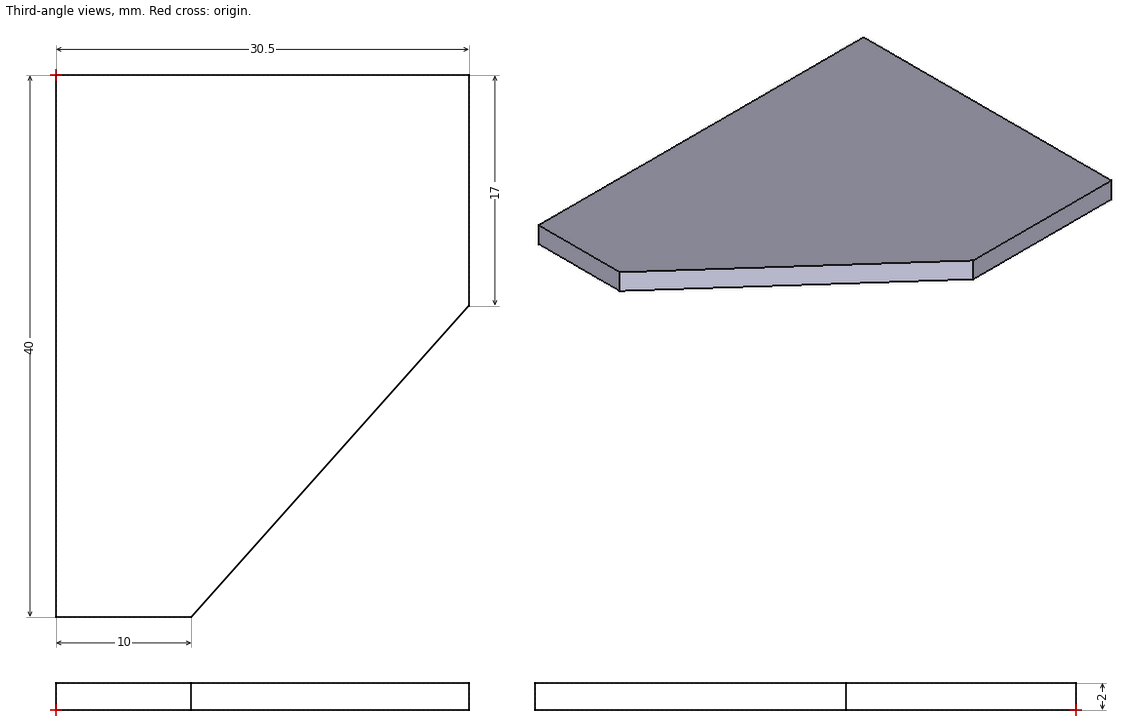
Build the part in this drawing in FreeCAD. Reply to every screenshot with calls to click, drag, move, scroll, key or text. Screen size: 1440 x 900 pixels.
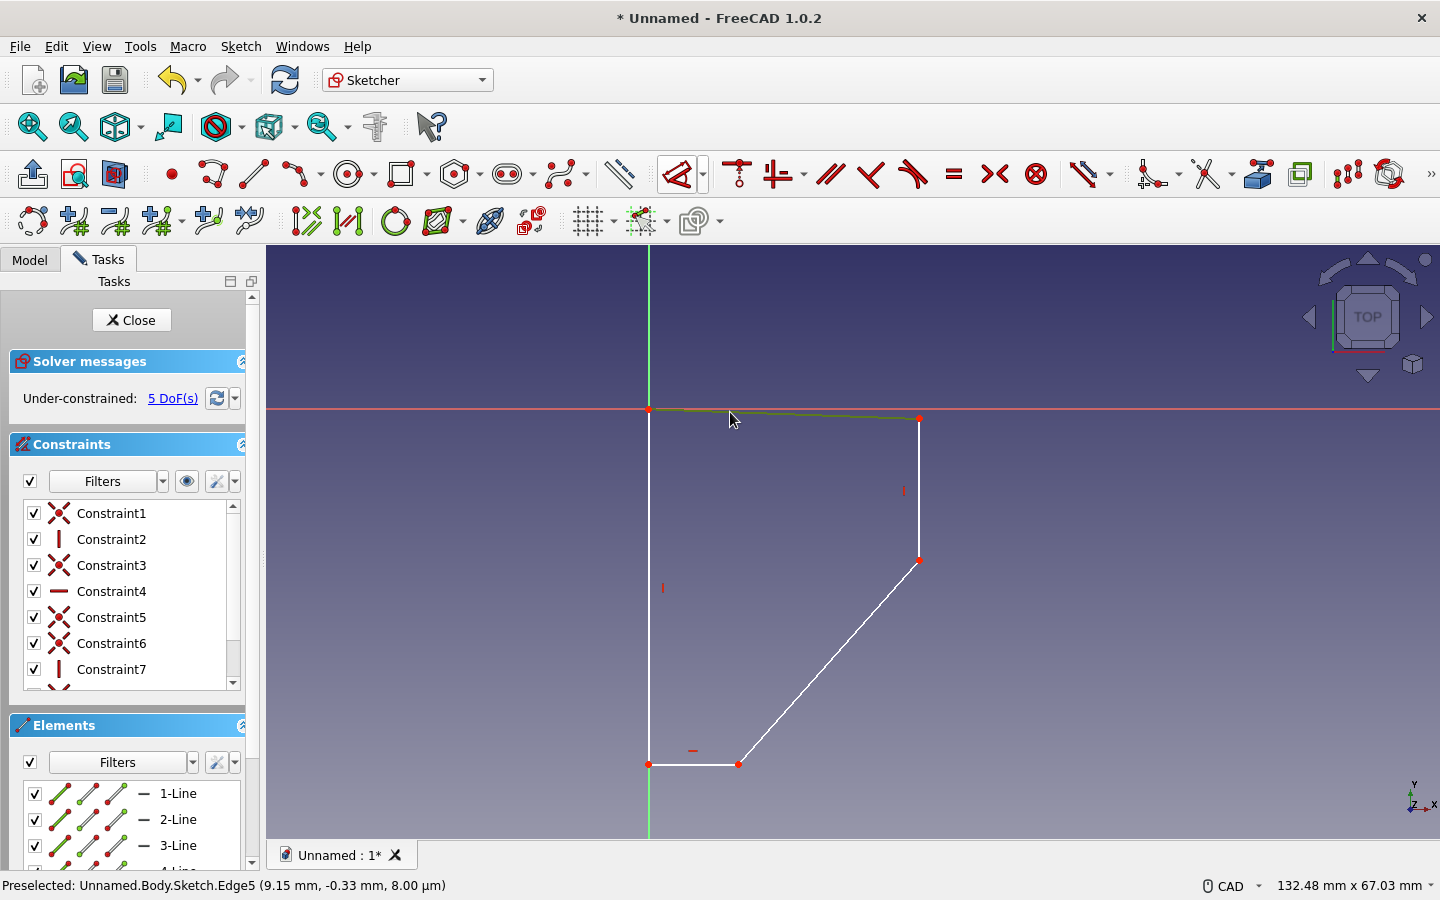
key(h)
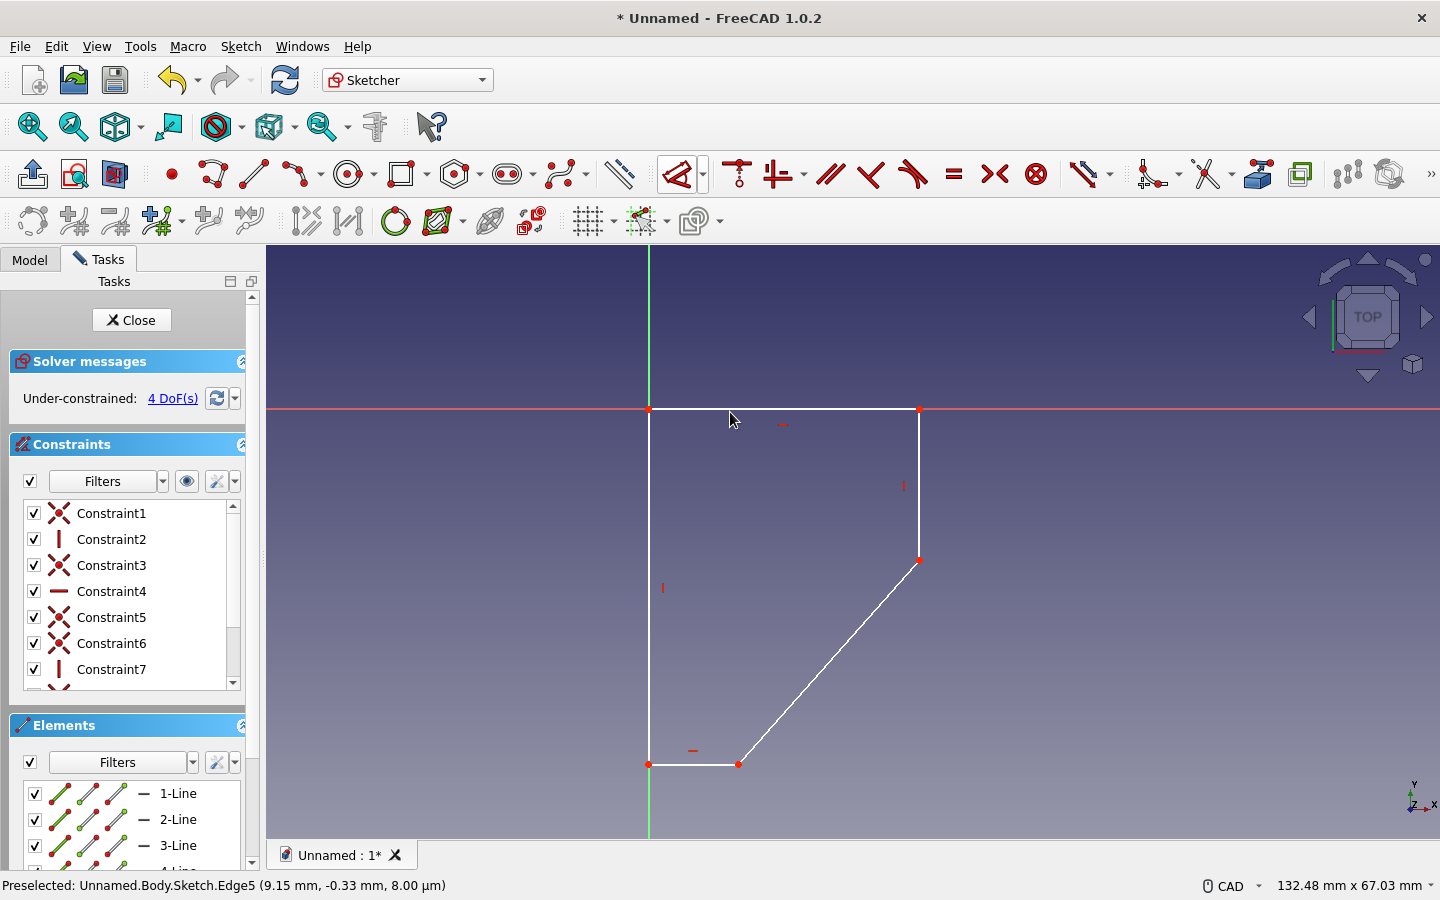
key(d)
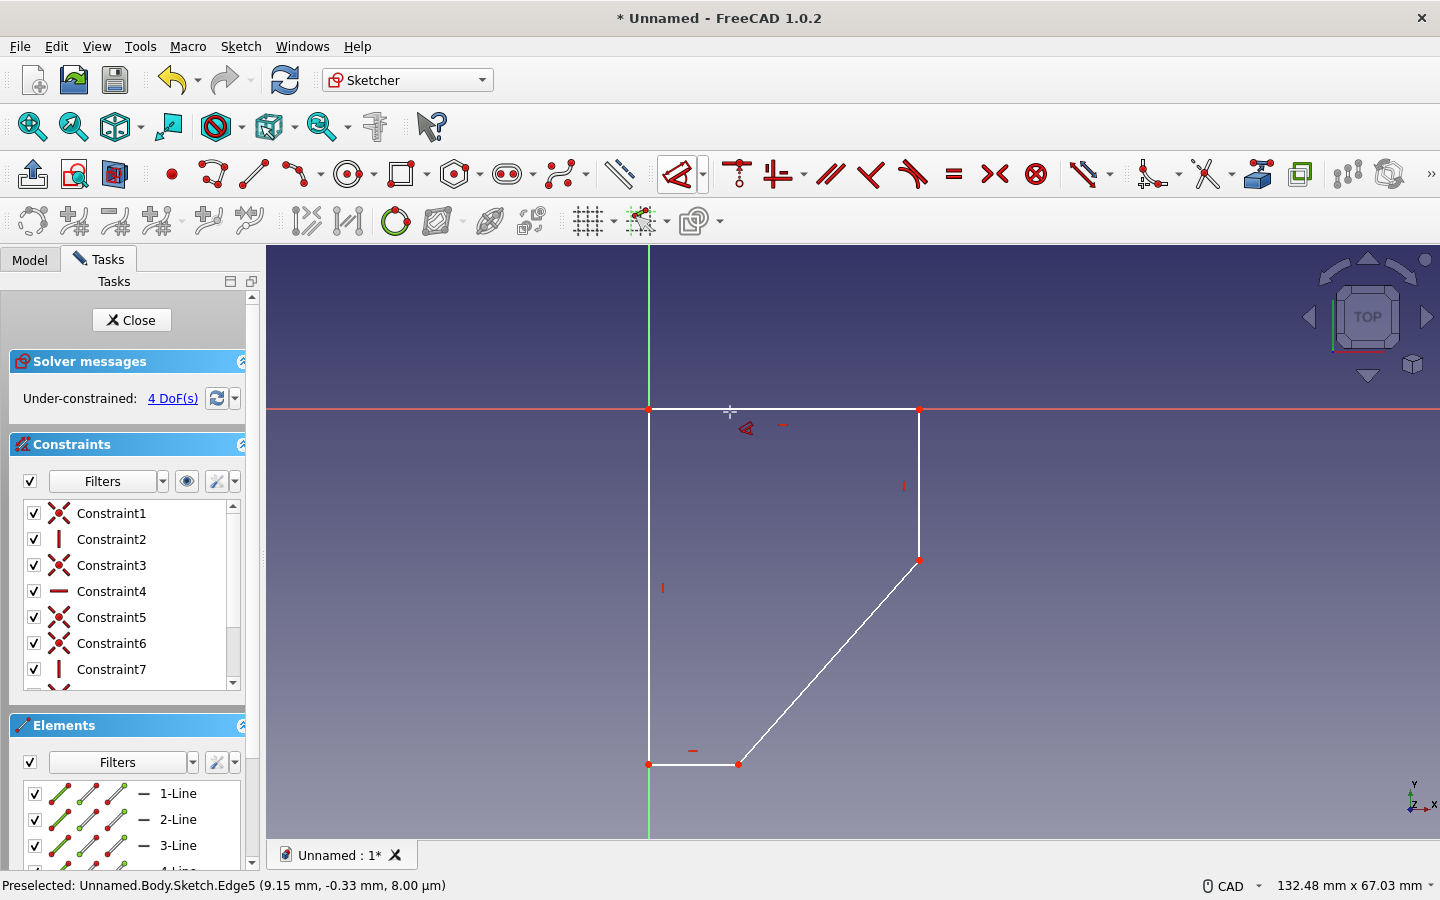
click(649, 516)
click(615, 587)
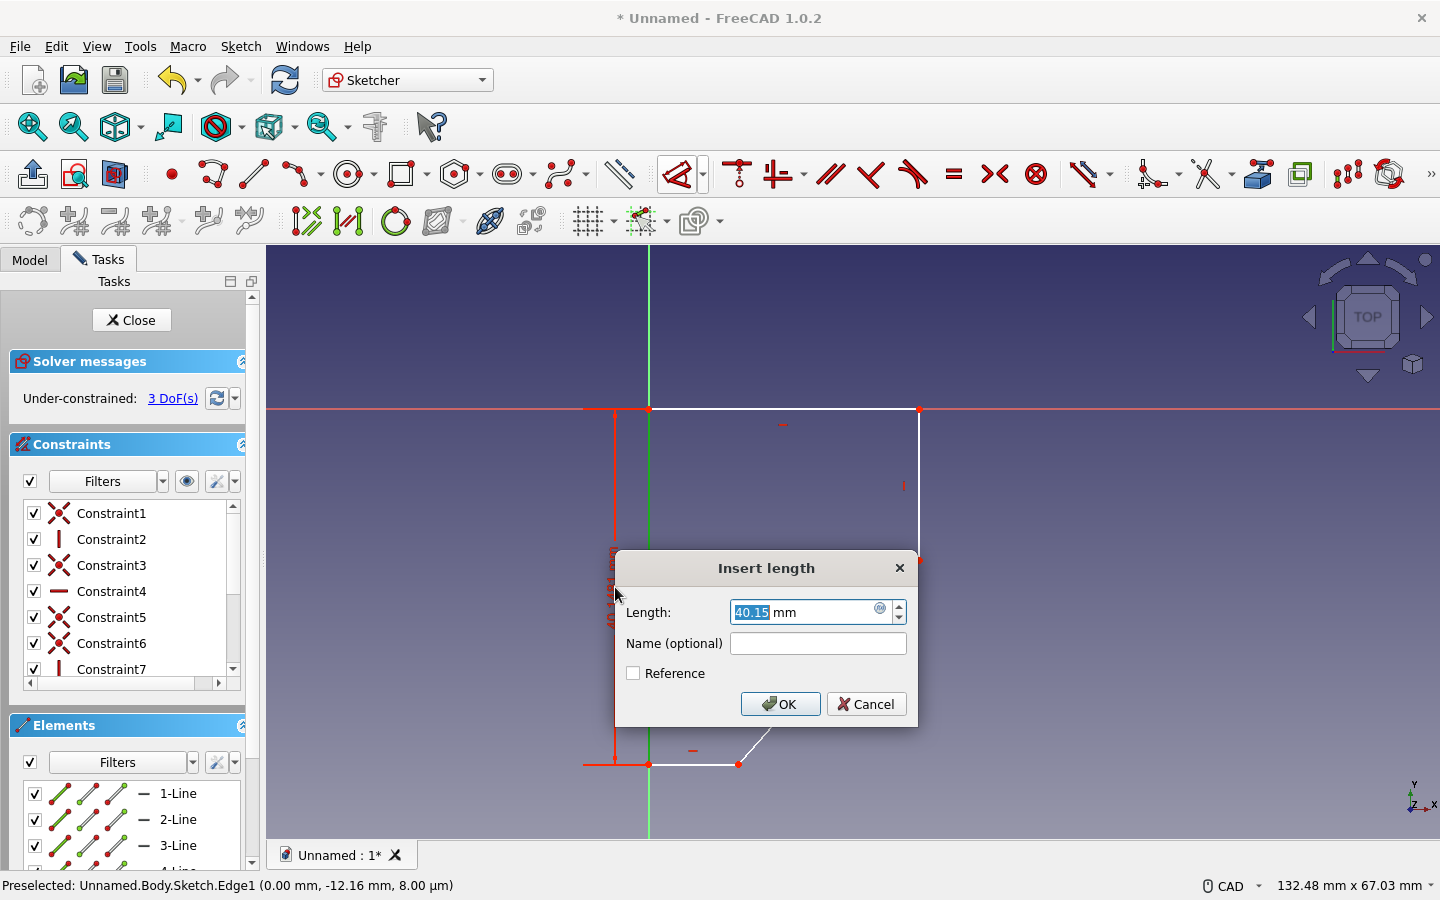
text(40)
key(Return)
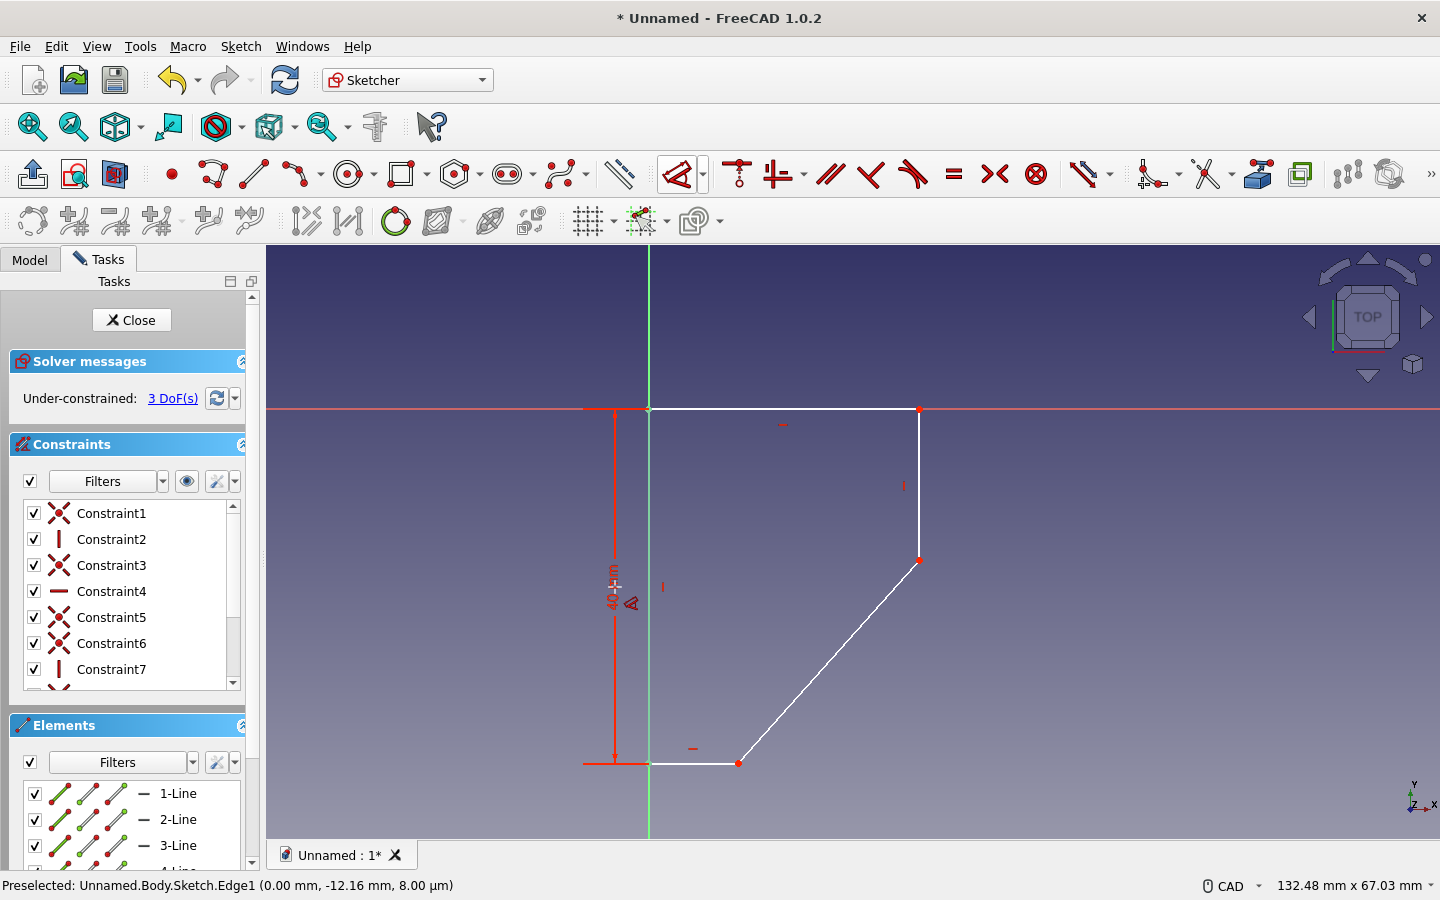
click(676, 764)
click(693, 798)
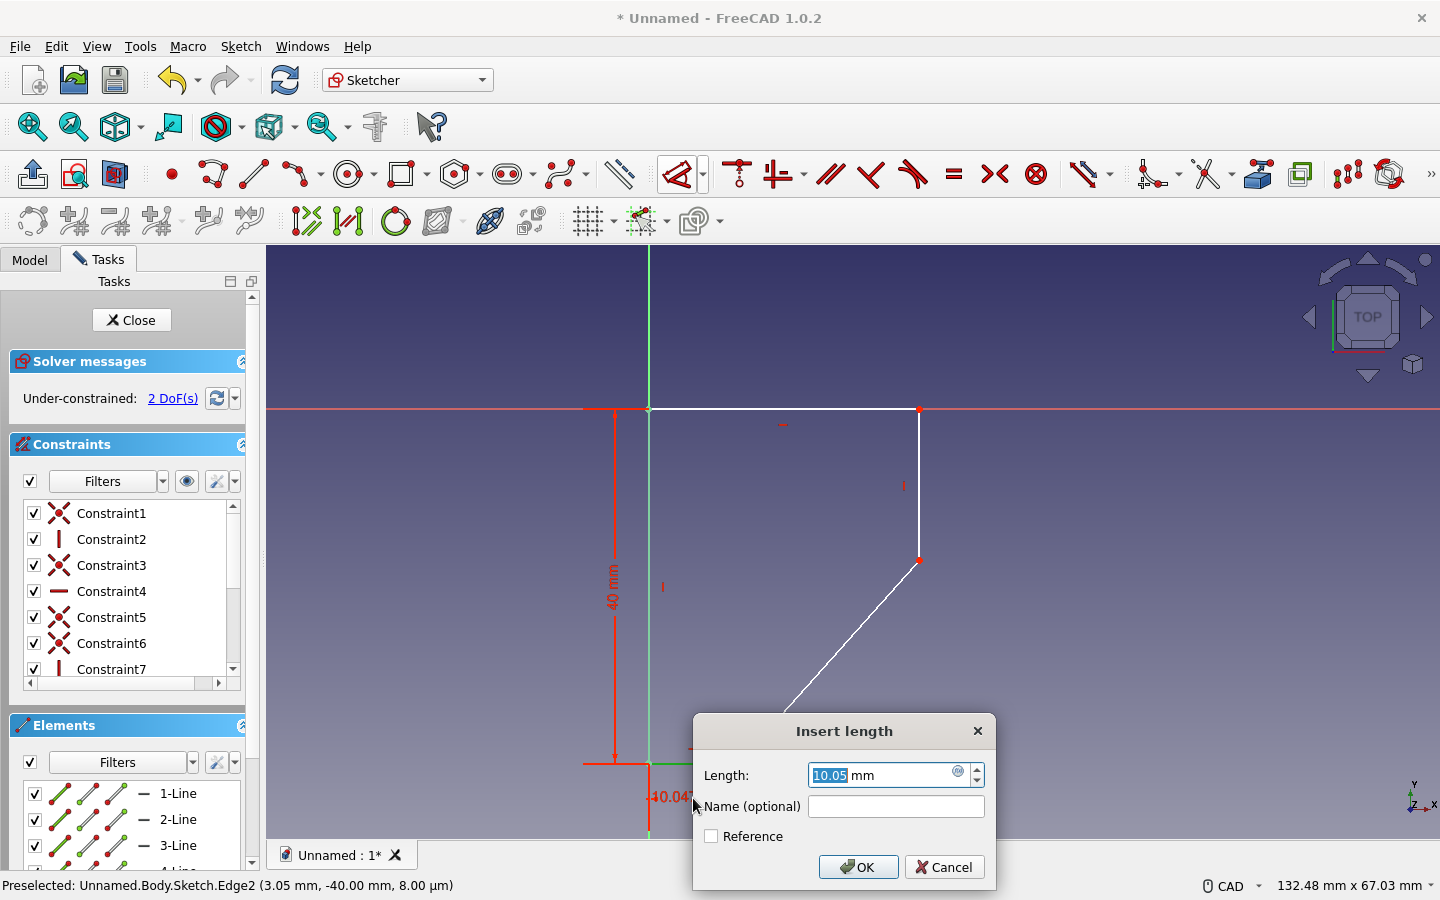
text(10)
key(Return)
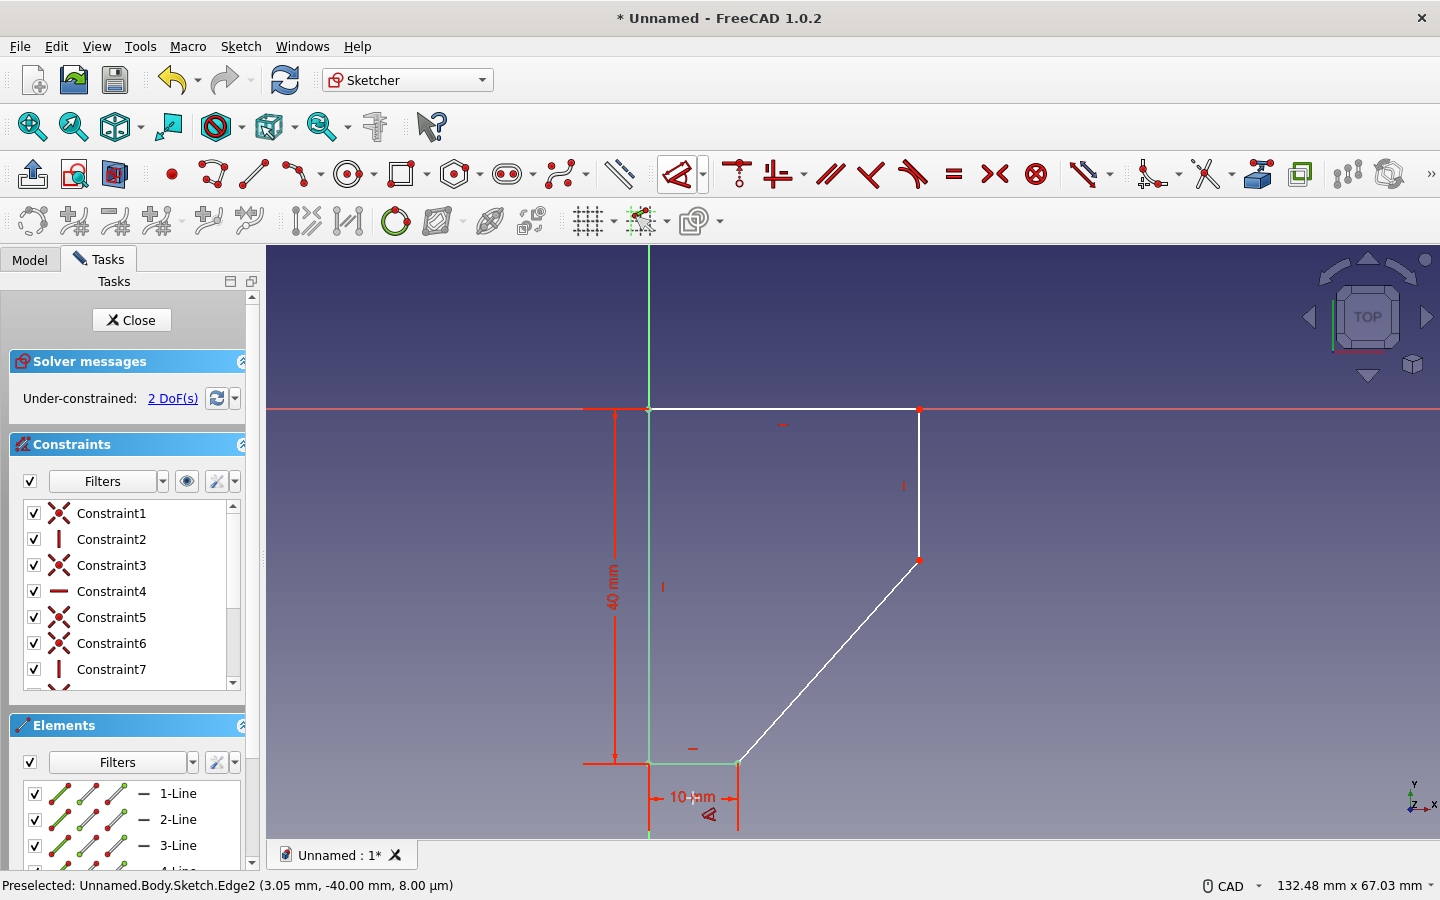
click(919, 515)
click(953, 485)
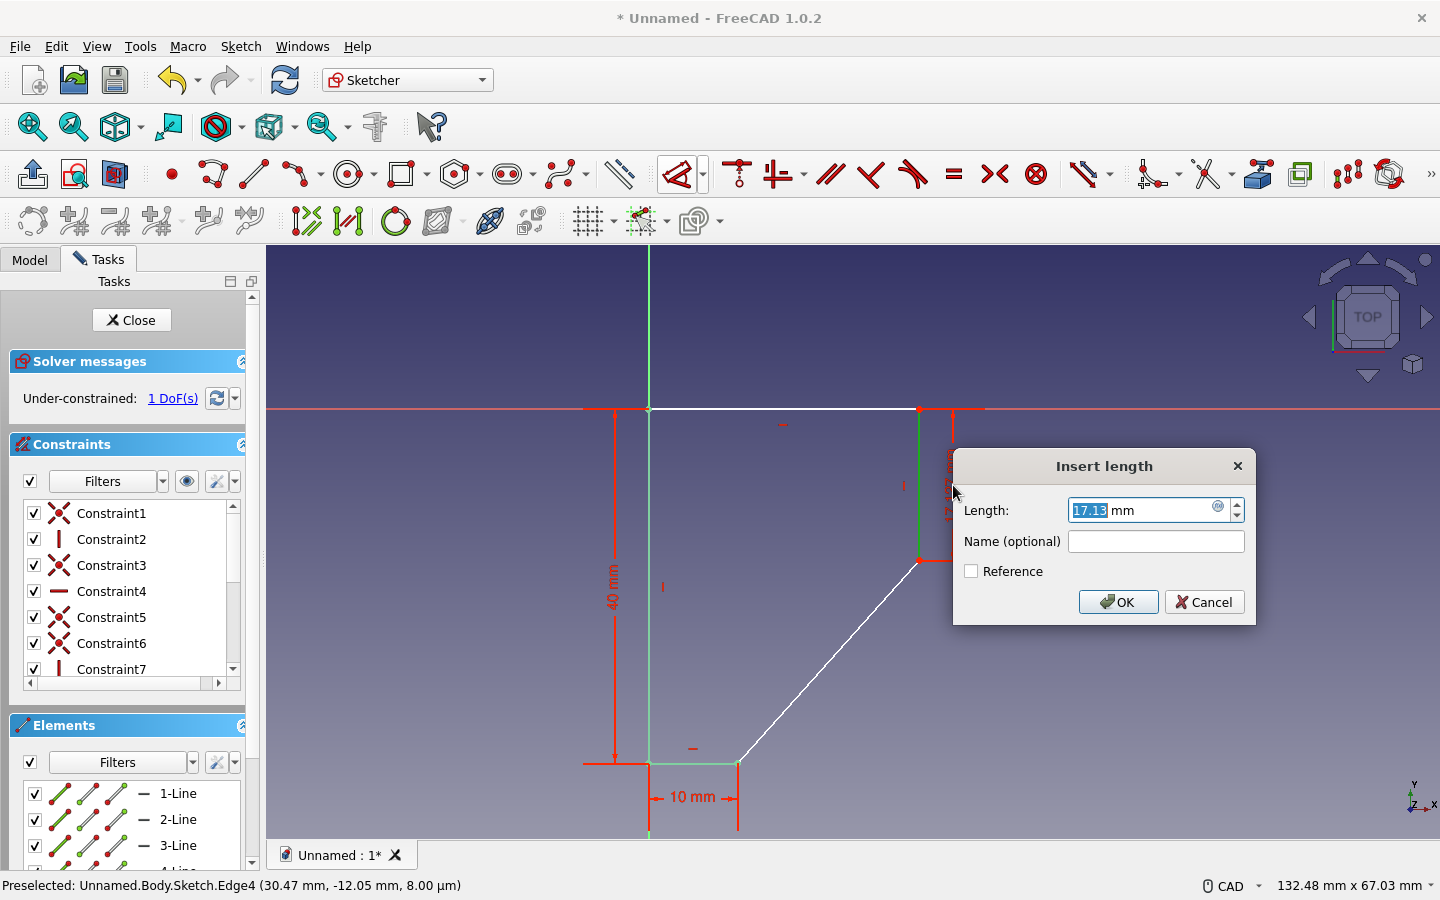
text(17)
key(Return)